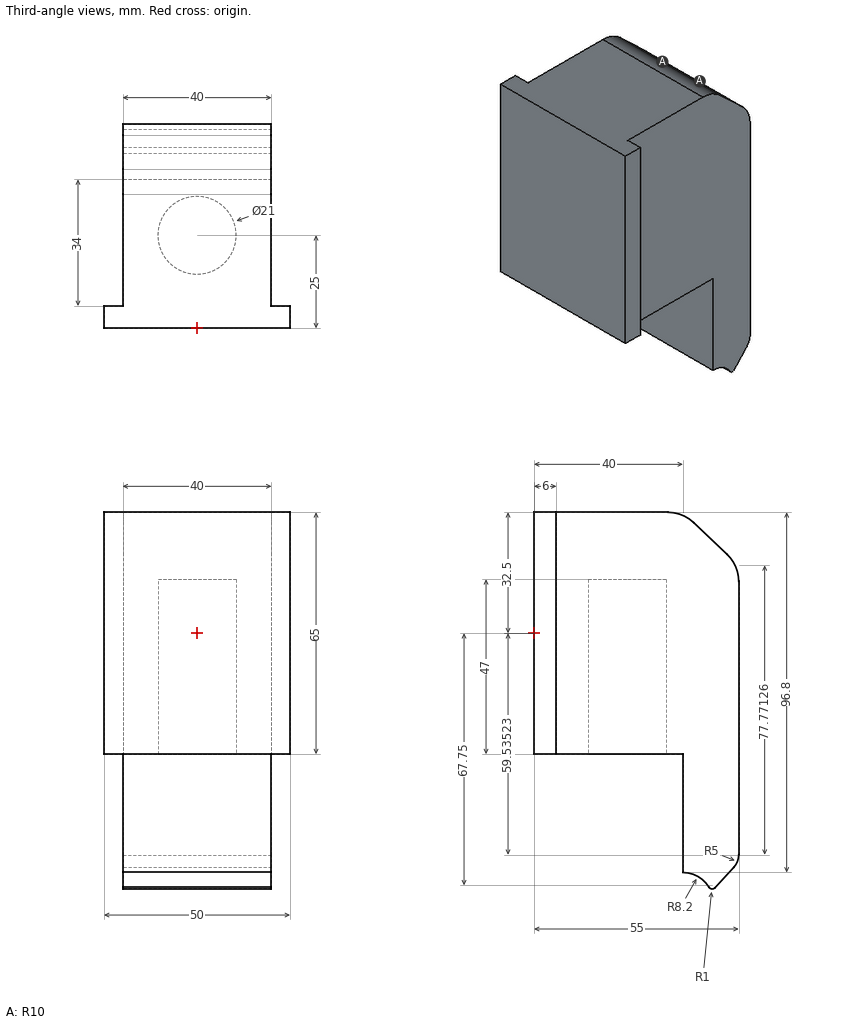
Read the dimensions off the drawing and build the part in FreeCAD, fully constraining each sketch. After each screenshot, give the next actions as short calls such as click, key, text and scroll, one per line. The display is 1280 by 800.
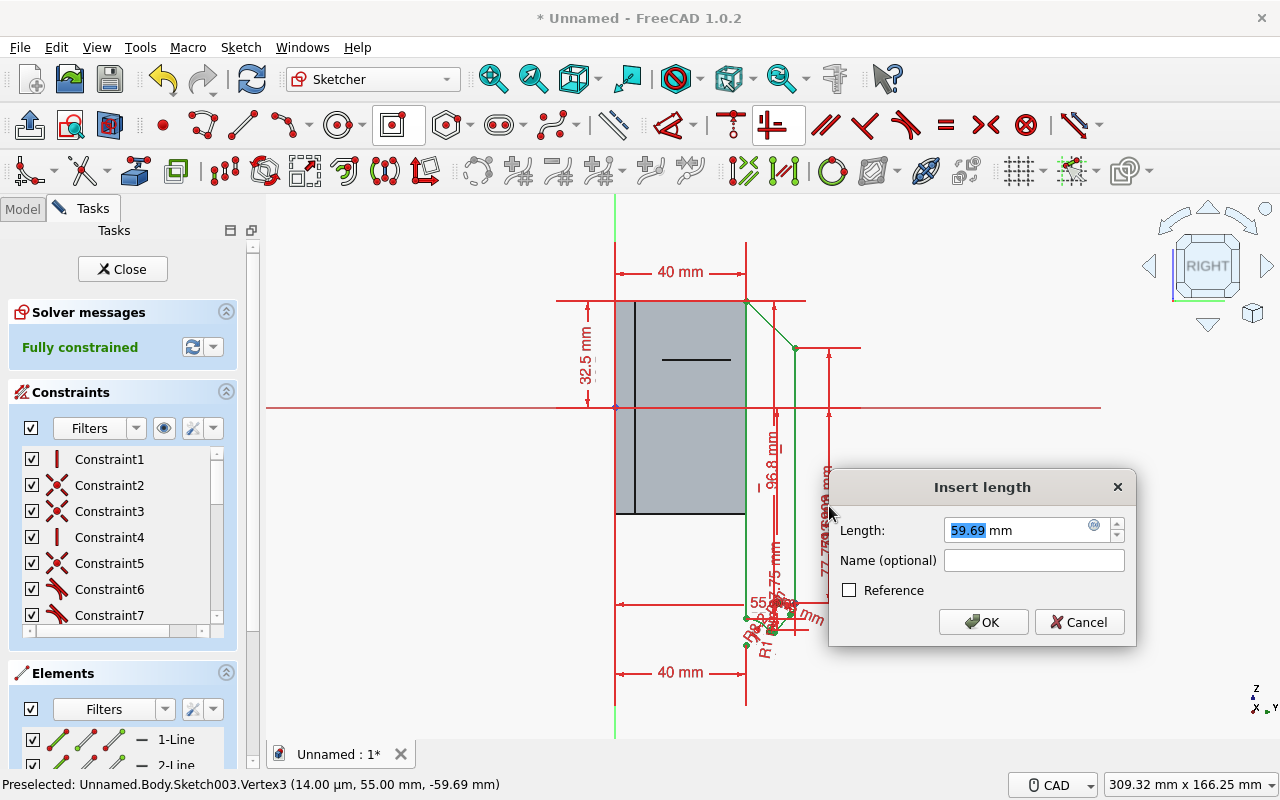
text(59.53523)
key(Return)
key(Escape)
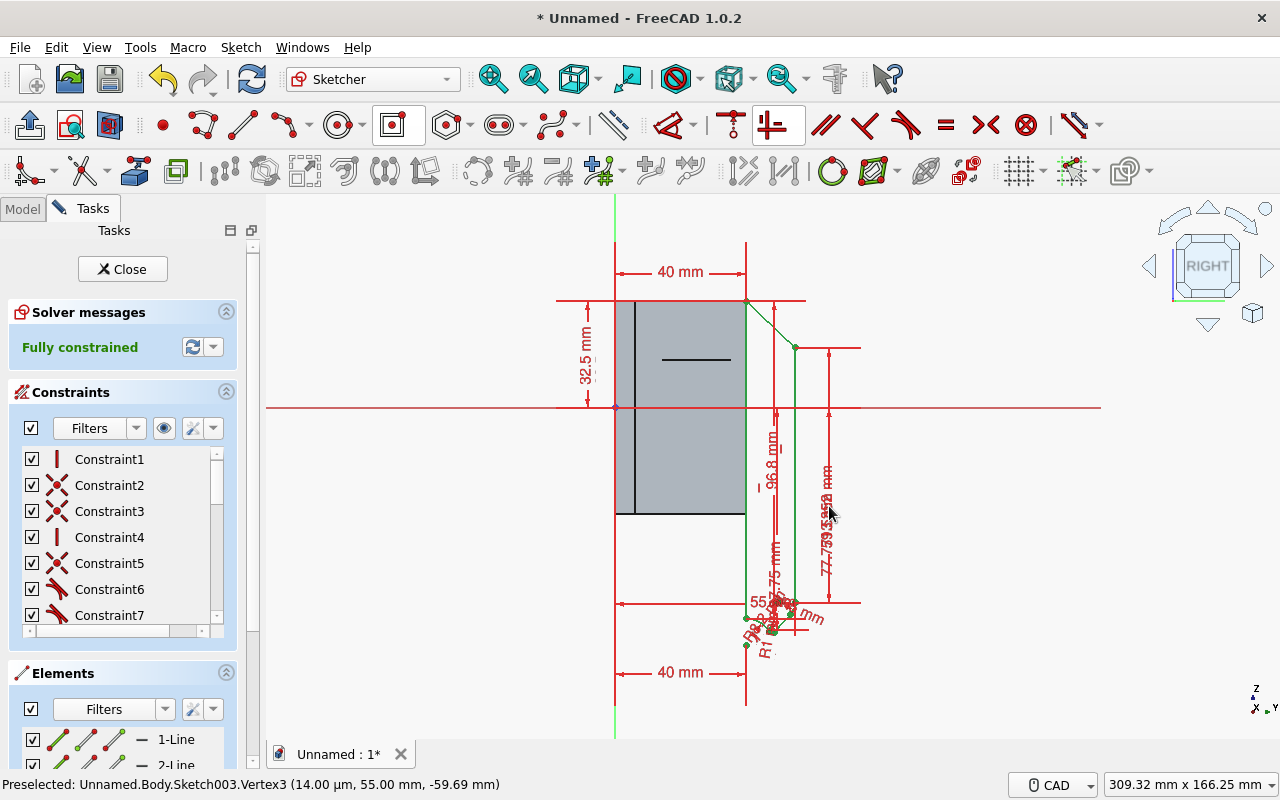
click(123, 269)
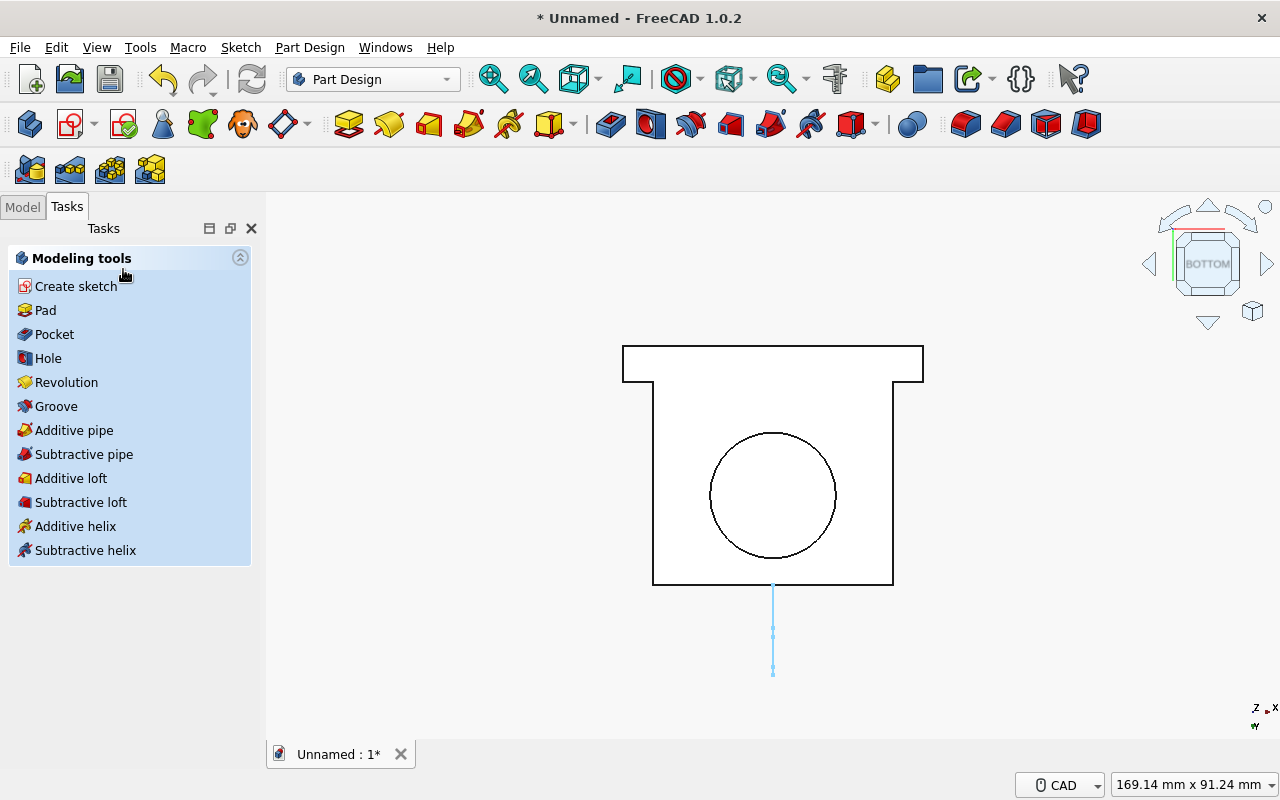
click(350, 124)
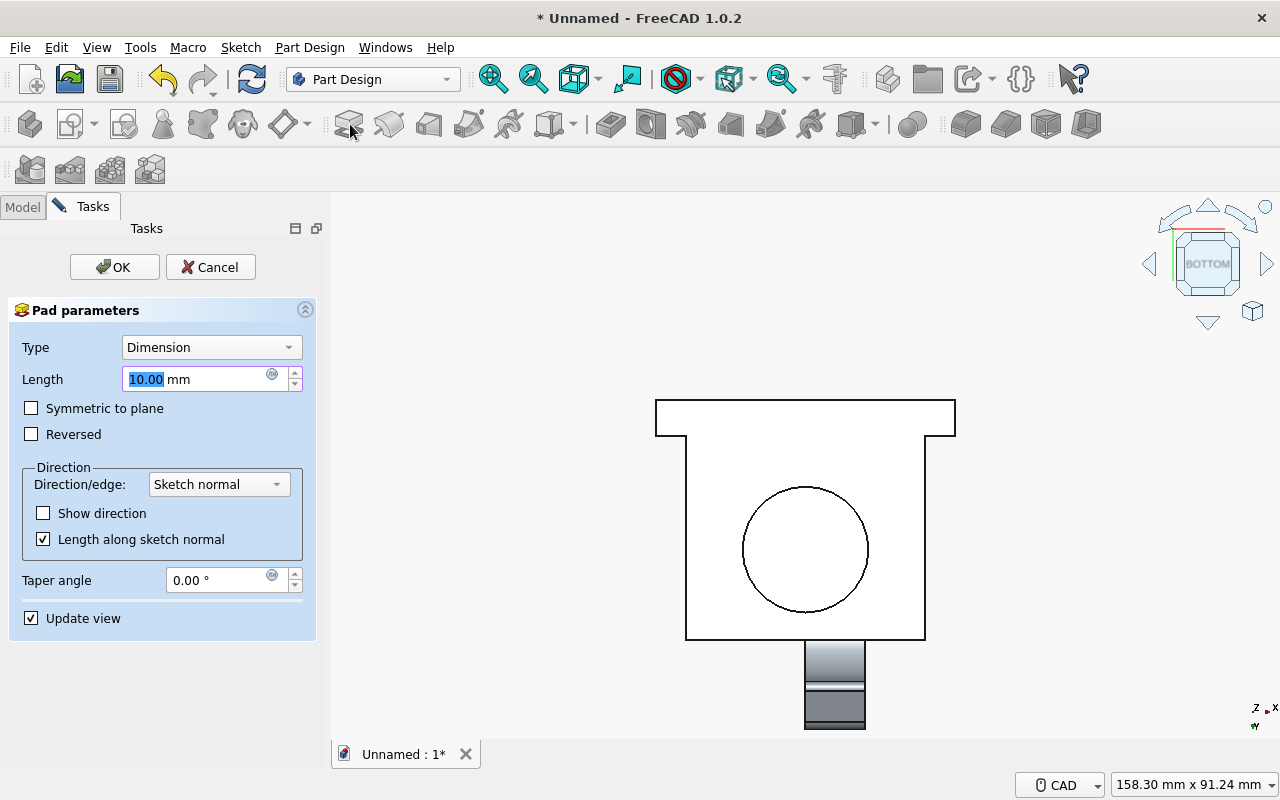
text(40)
key(Tab)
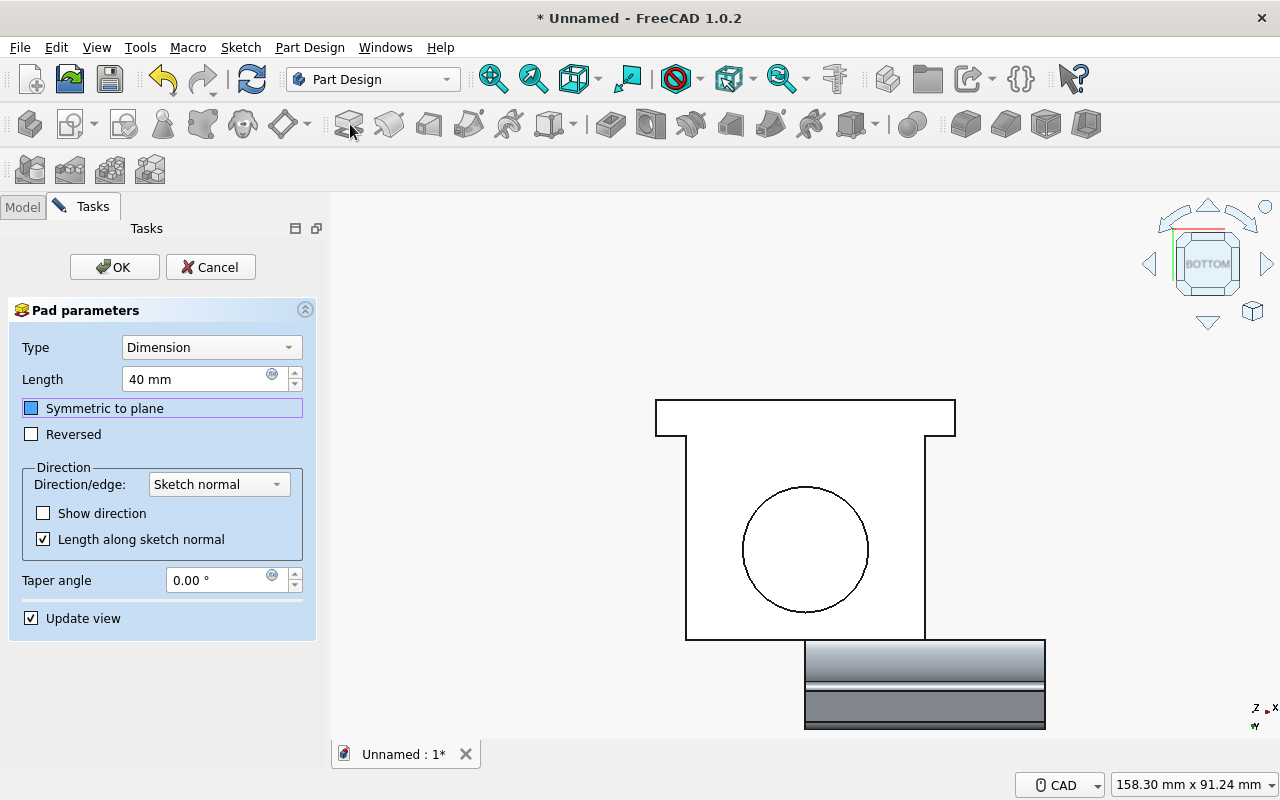
click(30, 408)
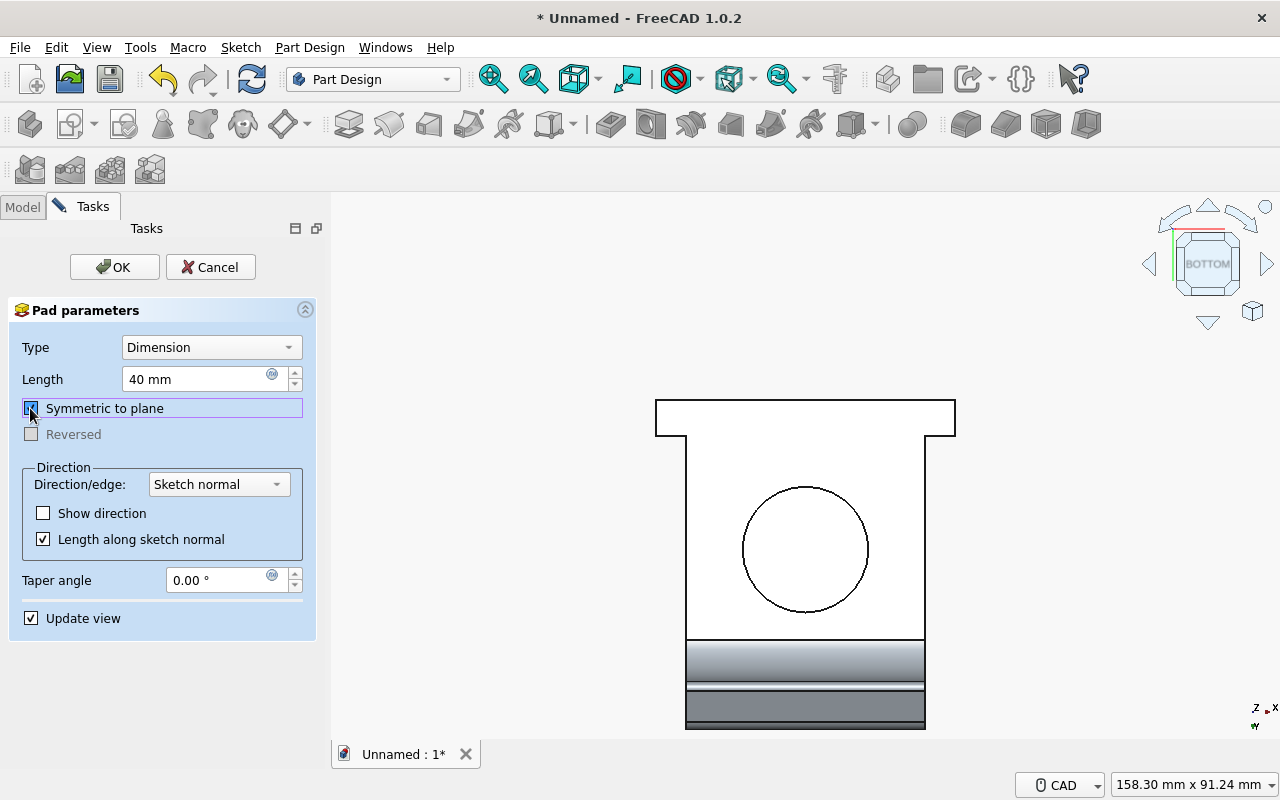
click(115, 267)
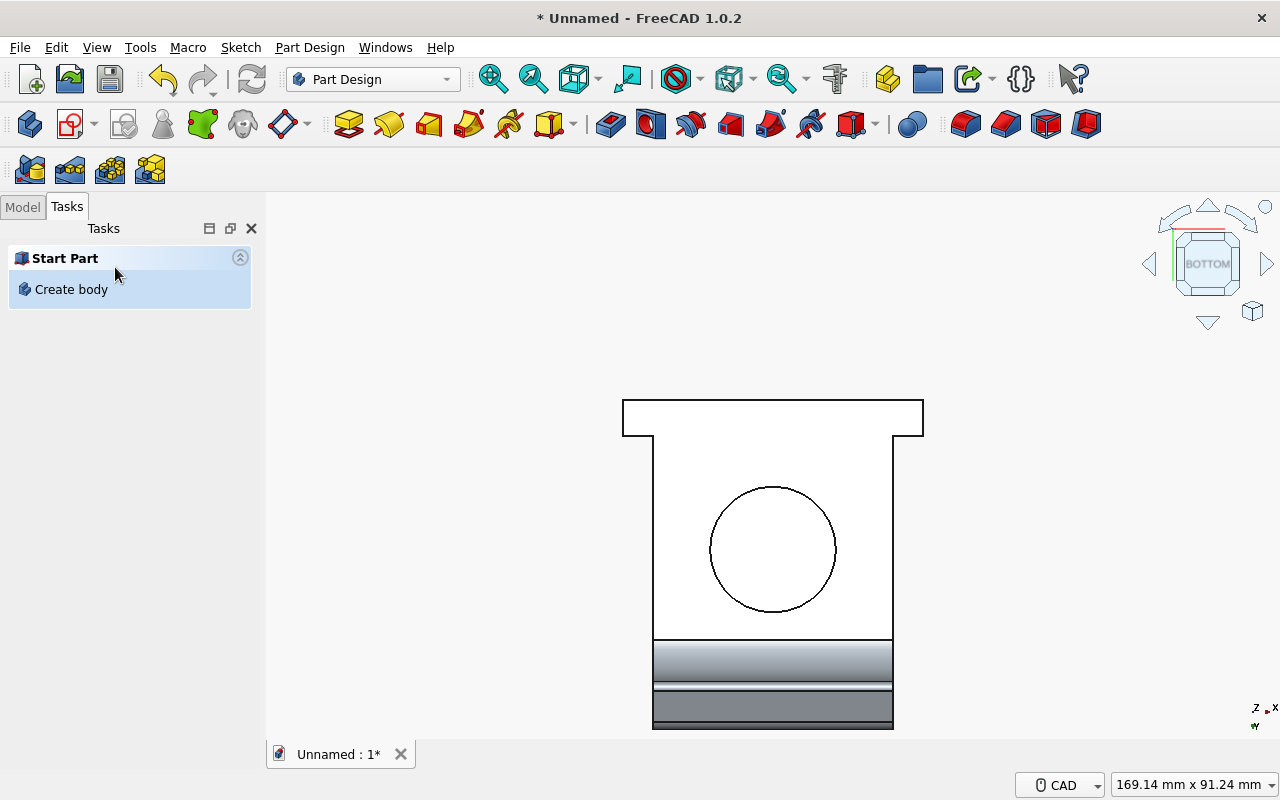
key(0)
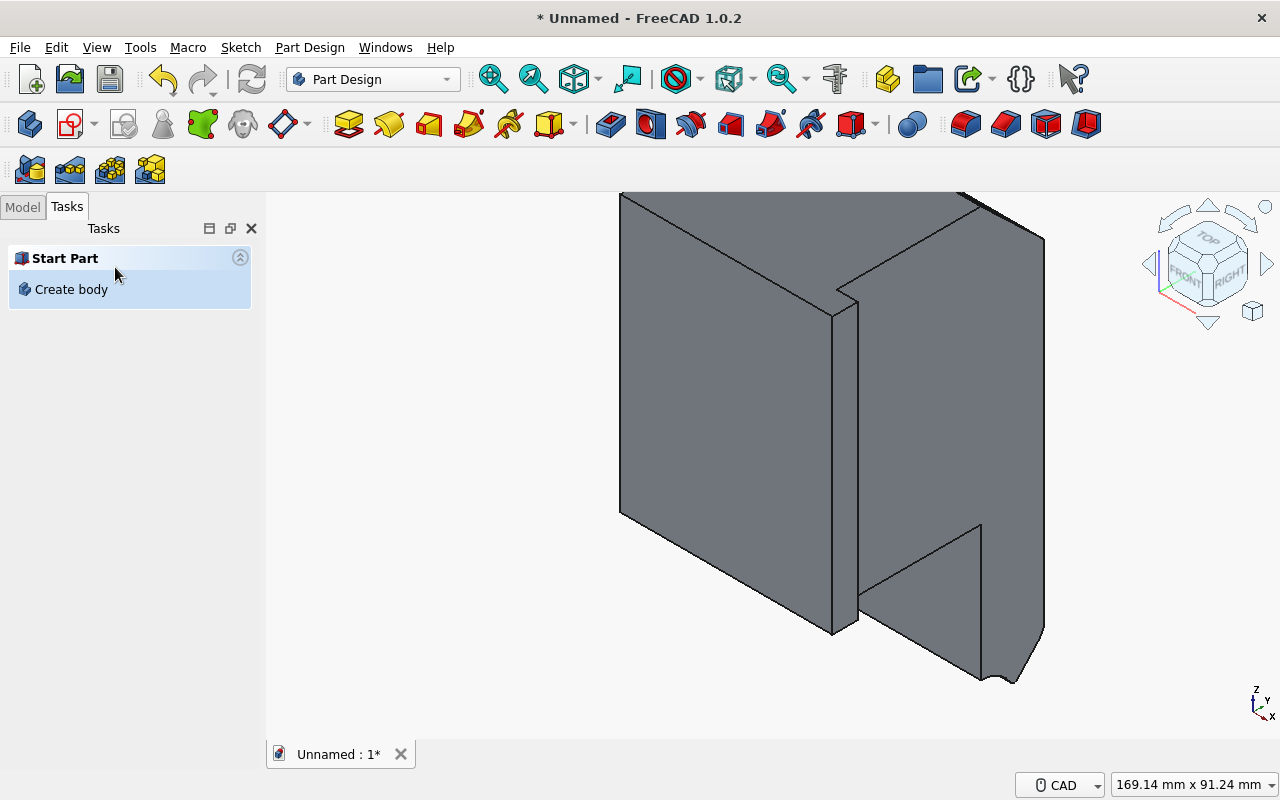
click(494, 80)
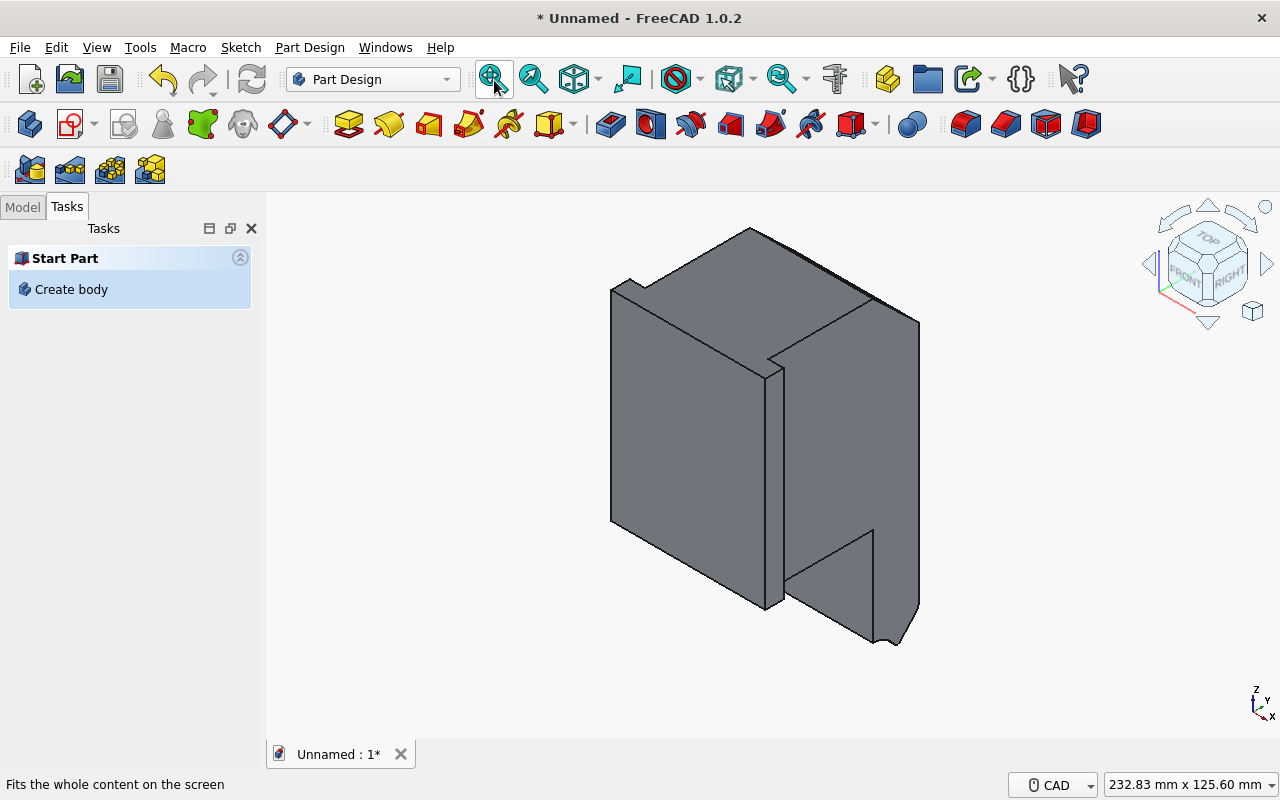
key(2)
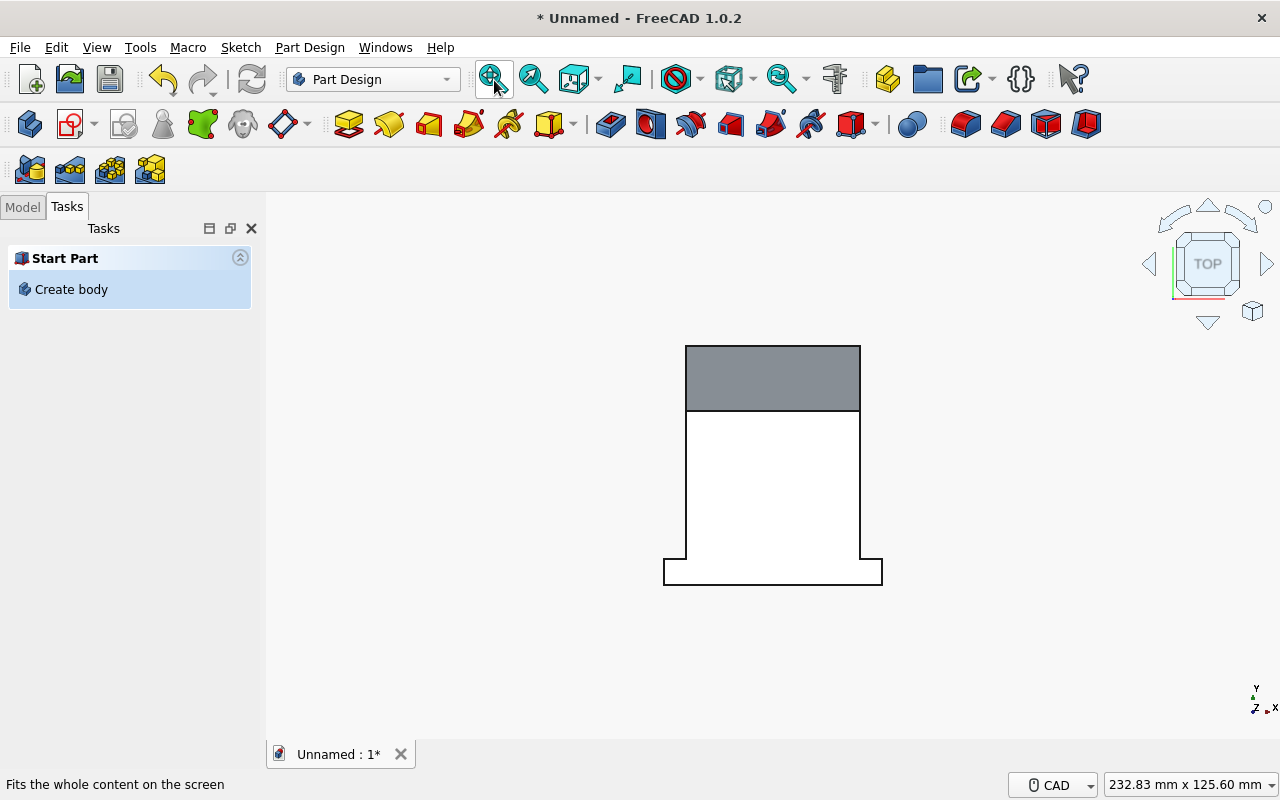
click(494, 80)